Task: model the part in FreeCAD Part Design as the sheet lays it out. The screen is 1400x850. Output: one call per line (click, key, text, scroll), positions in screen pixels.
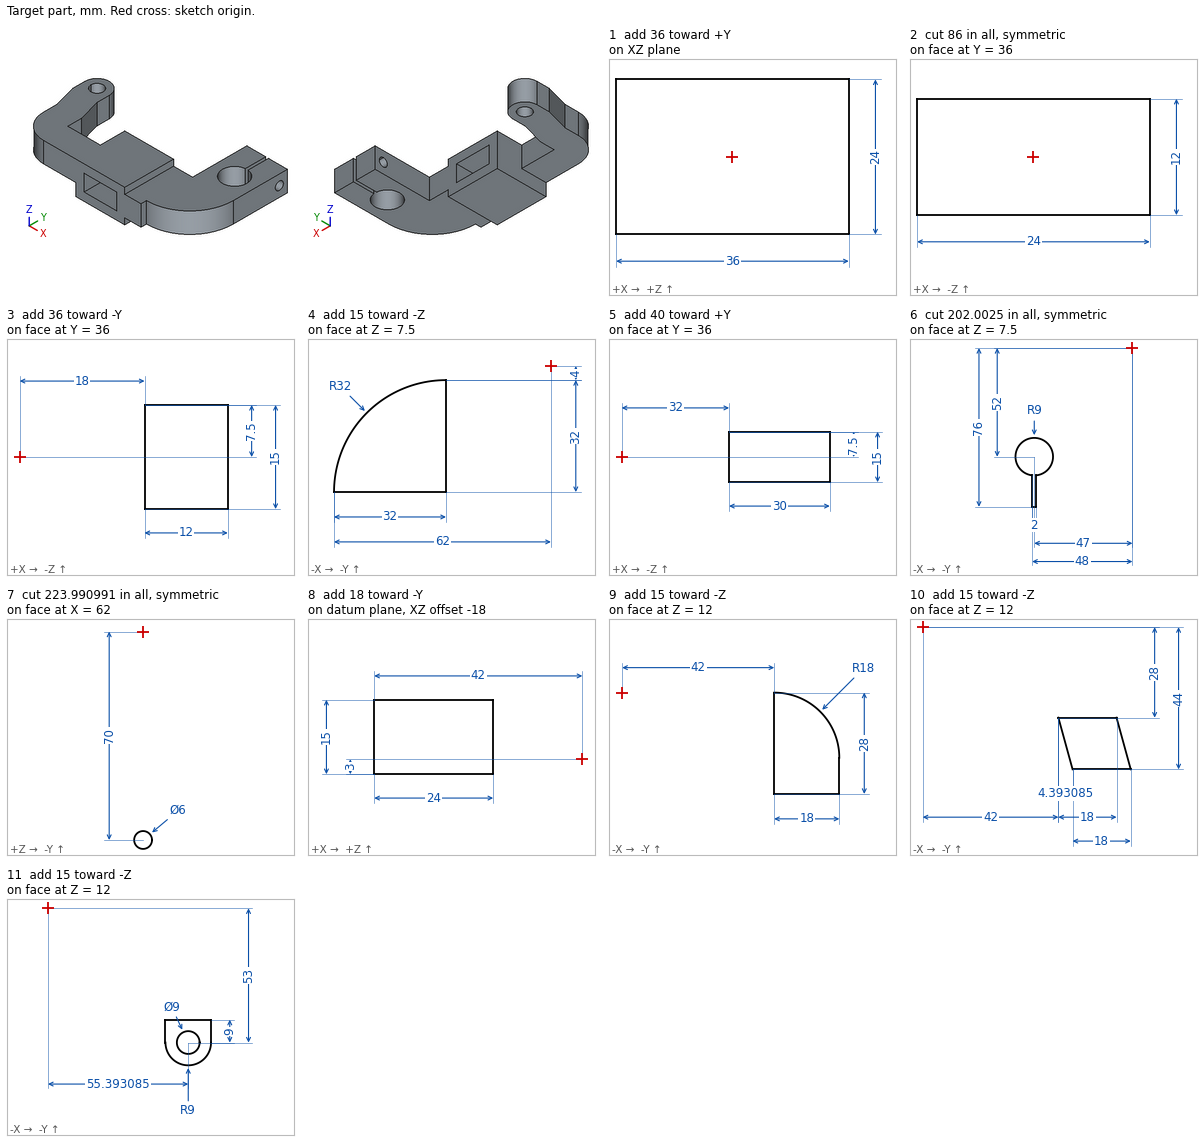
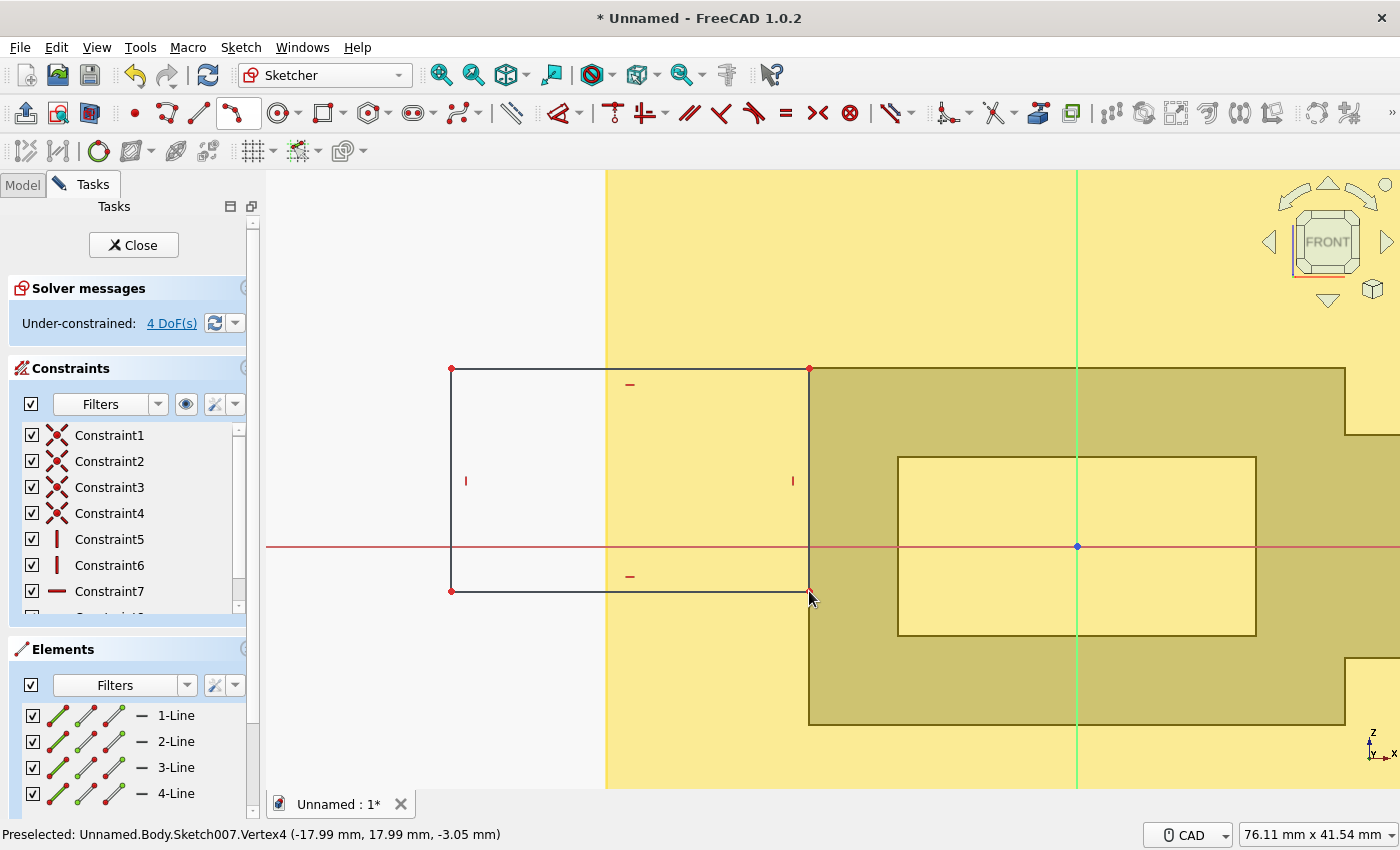
key(d)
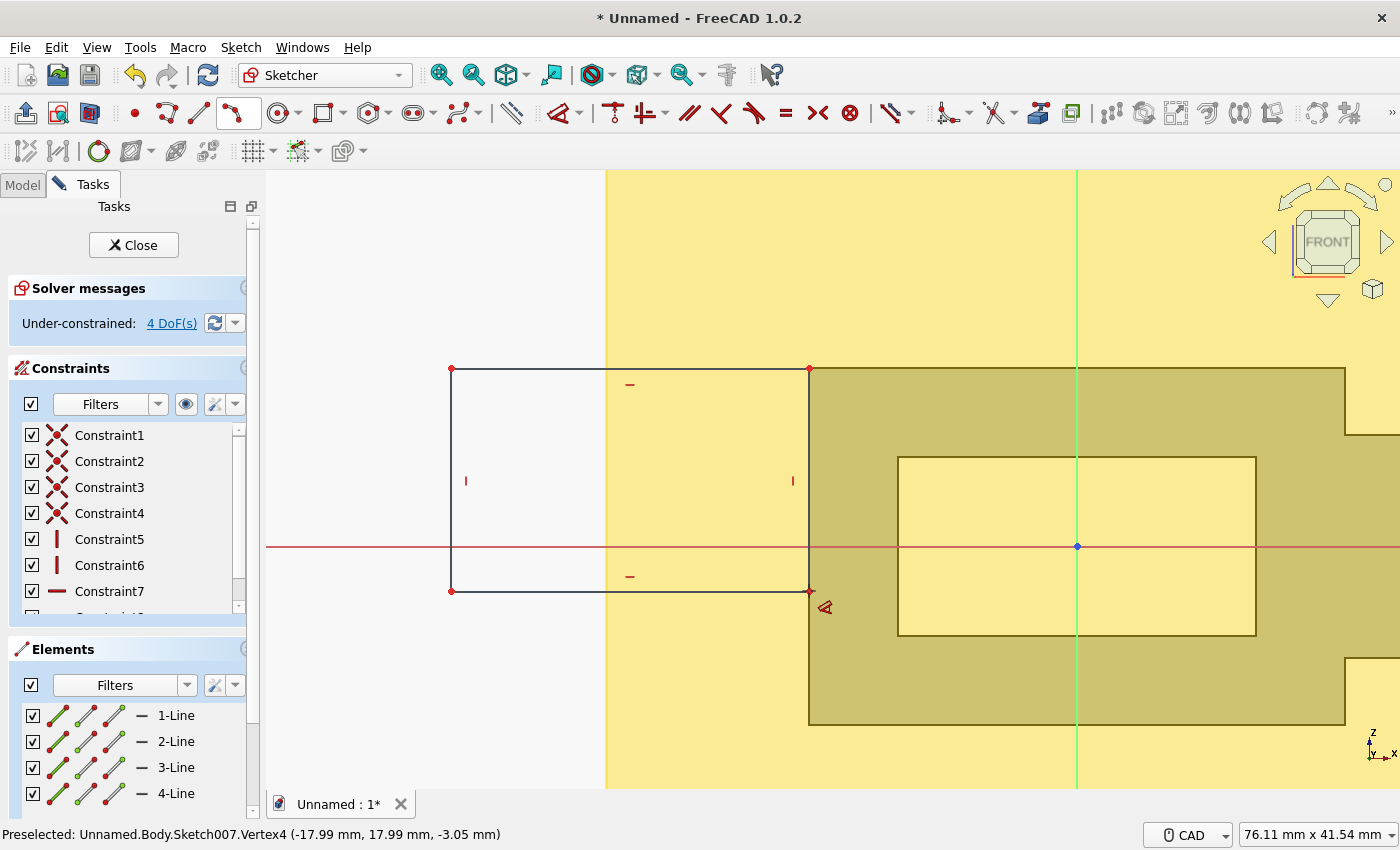
click(451, 436)
click(417, 481)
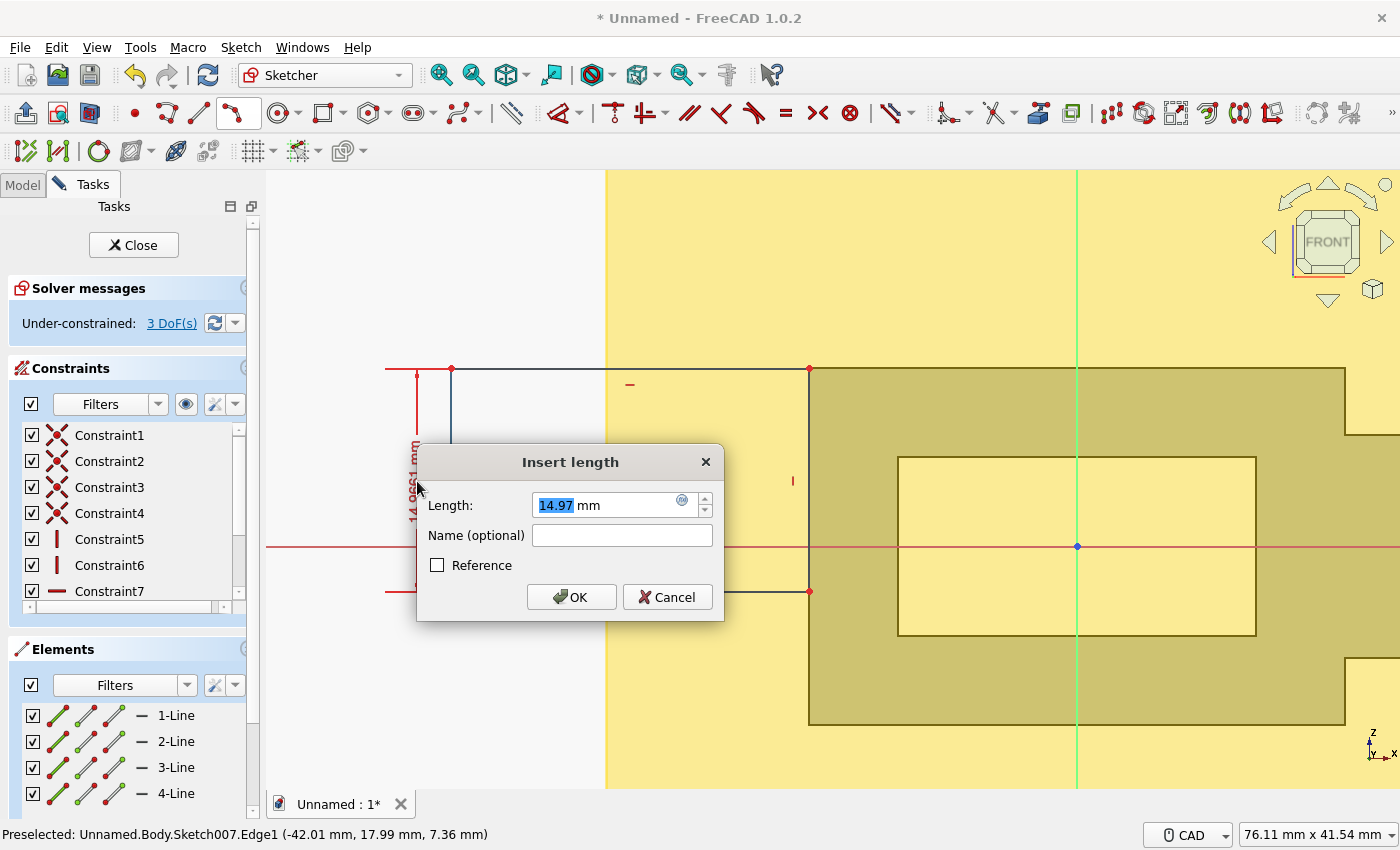
text(15)
key(Return)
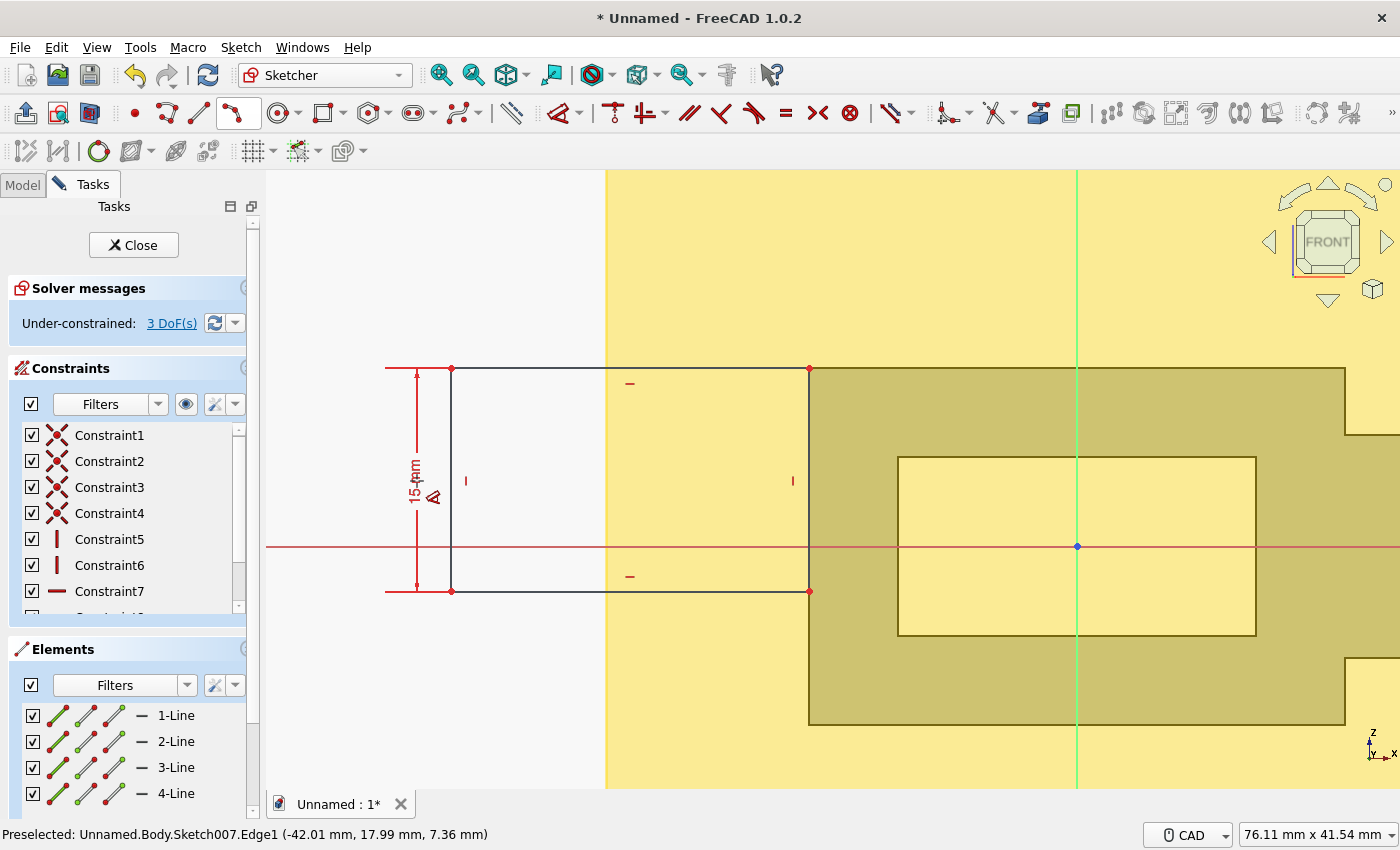
click(558, 592)
click(630, 626)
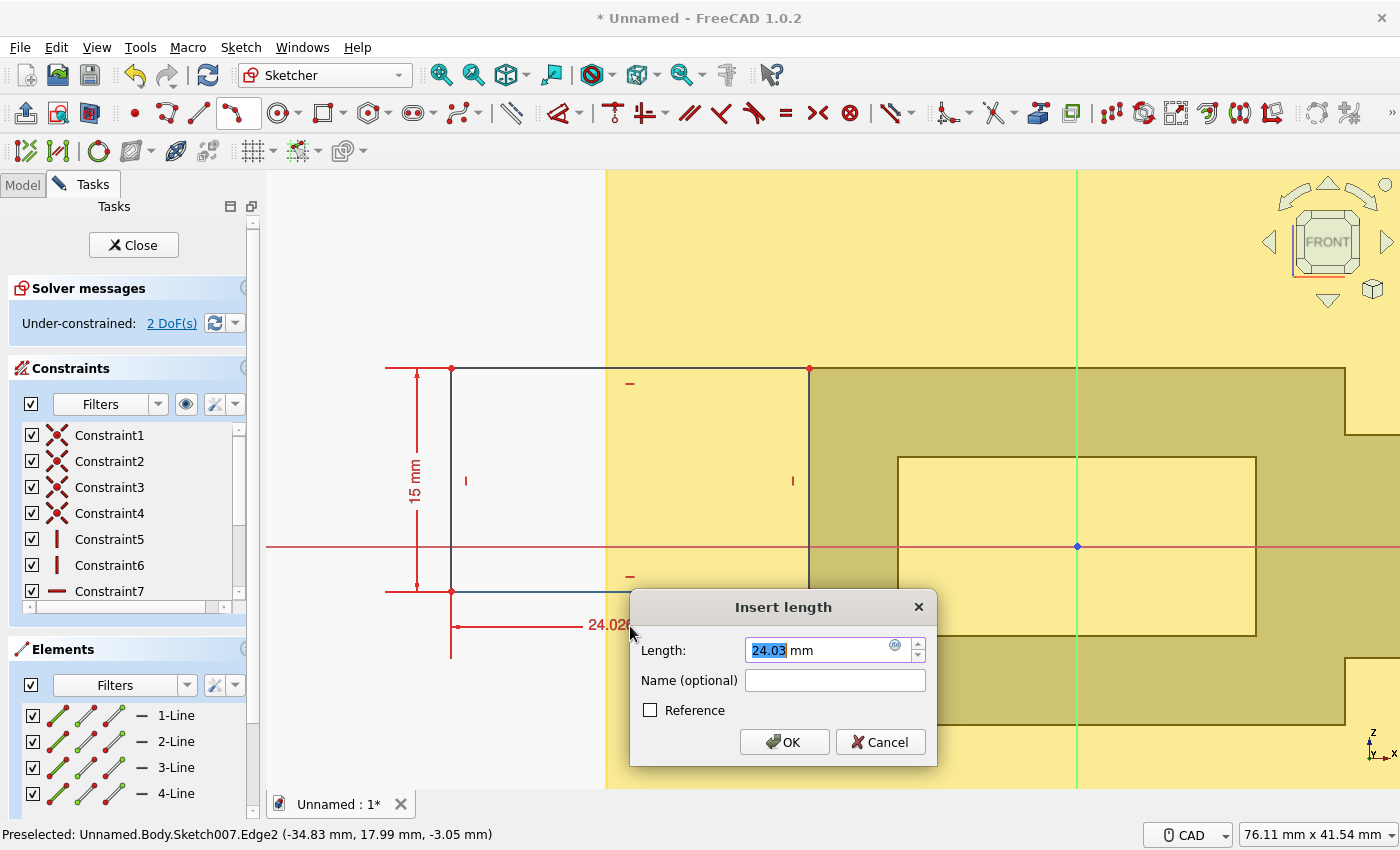
text(24)
key(Return)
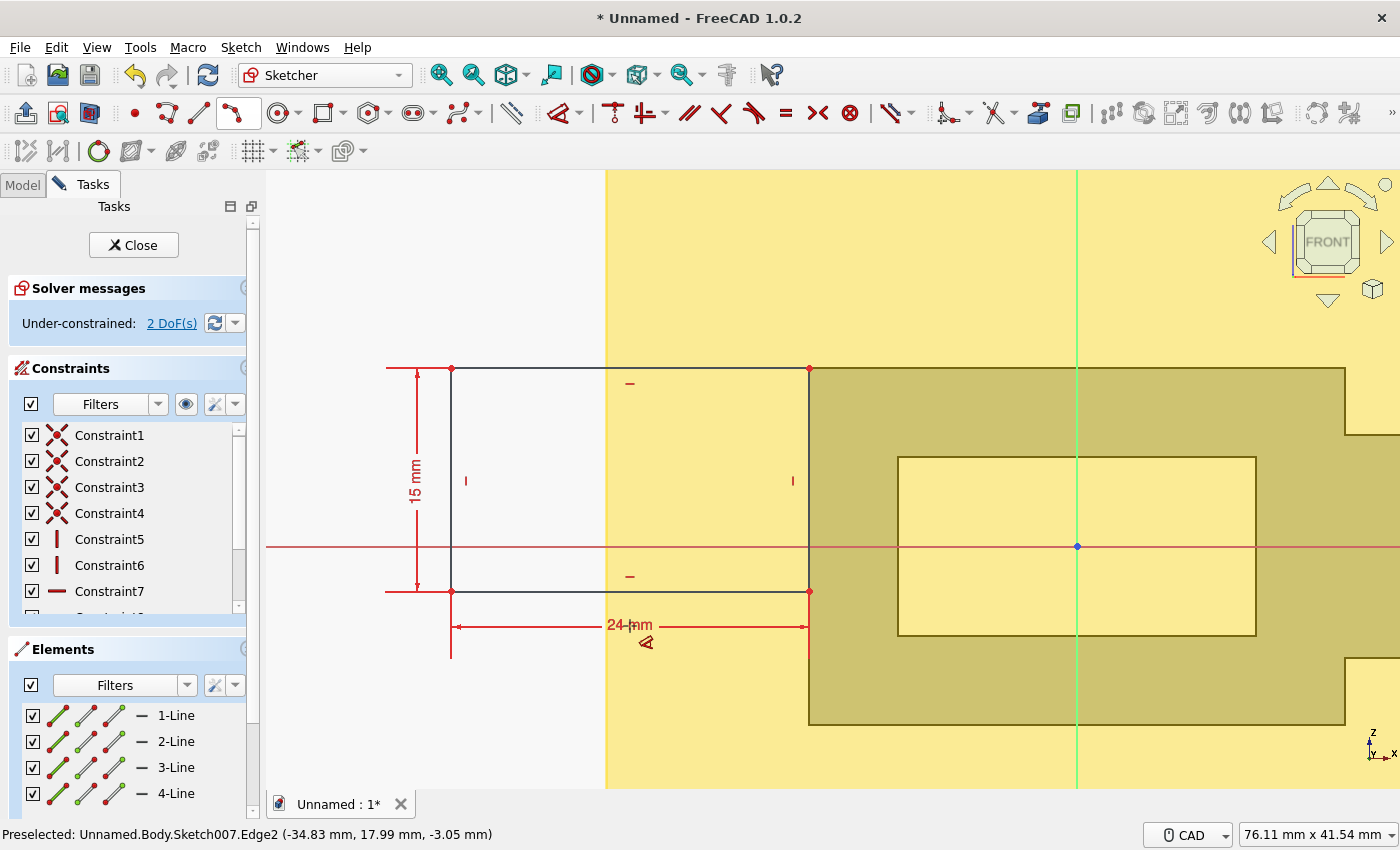
click(451, 592)
click(1111, 569)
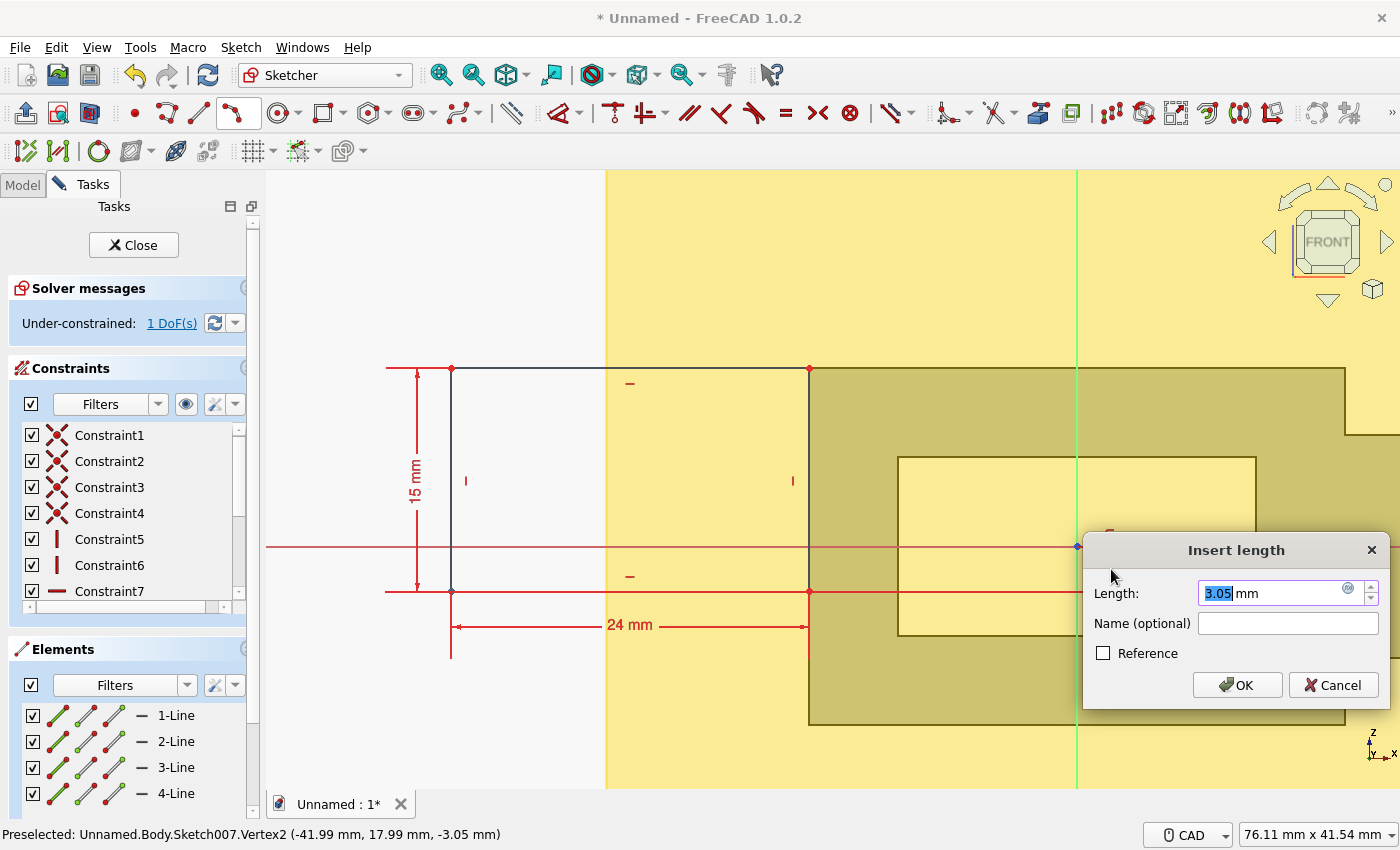
text(3)
key(Return)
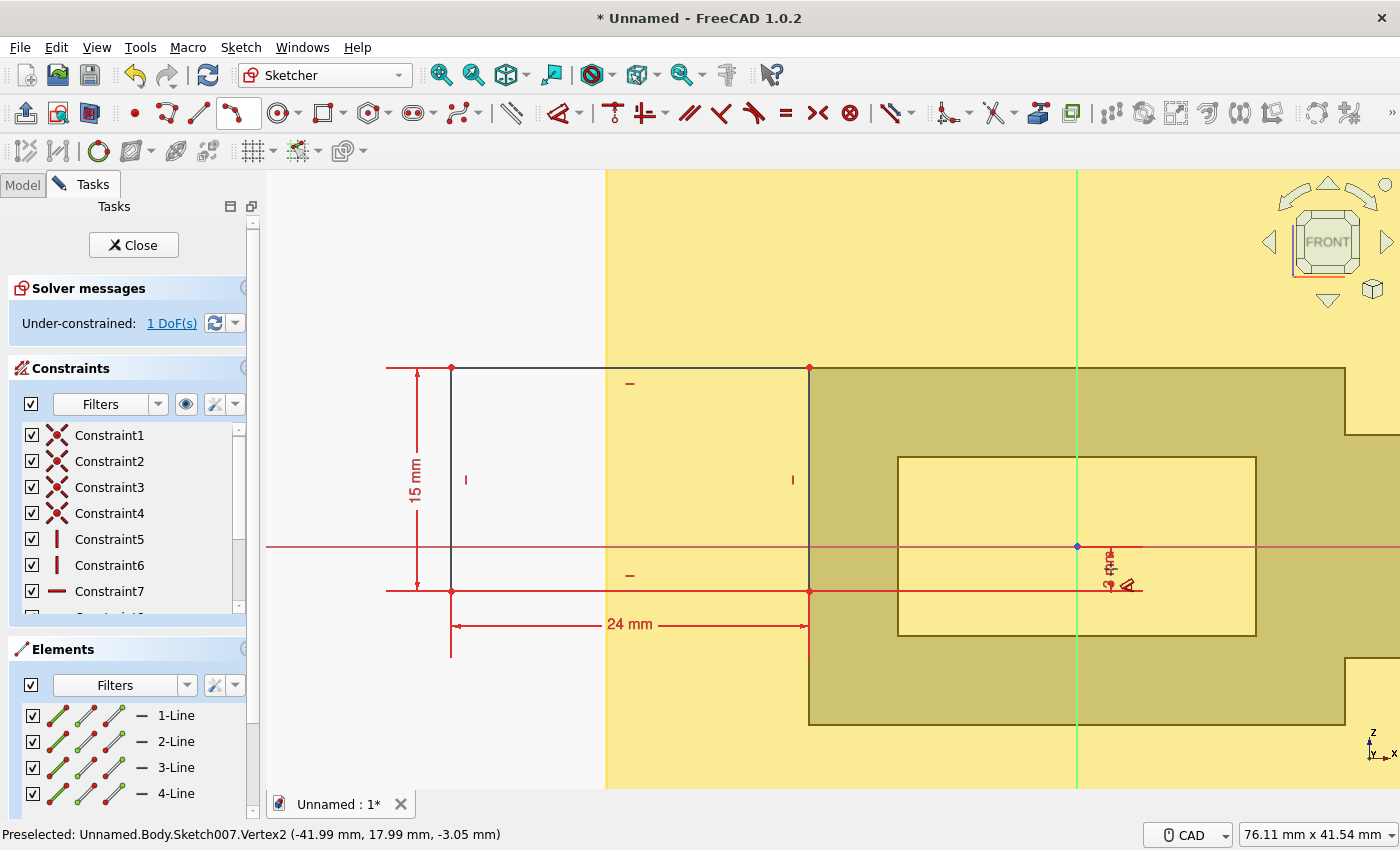
click(451, 368)
click(764, 334)